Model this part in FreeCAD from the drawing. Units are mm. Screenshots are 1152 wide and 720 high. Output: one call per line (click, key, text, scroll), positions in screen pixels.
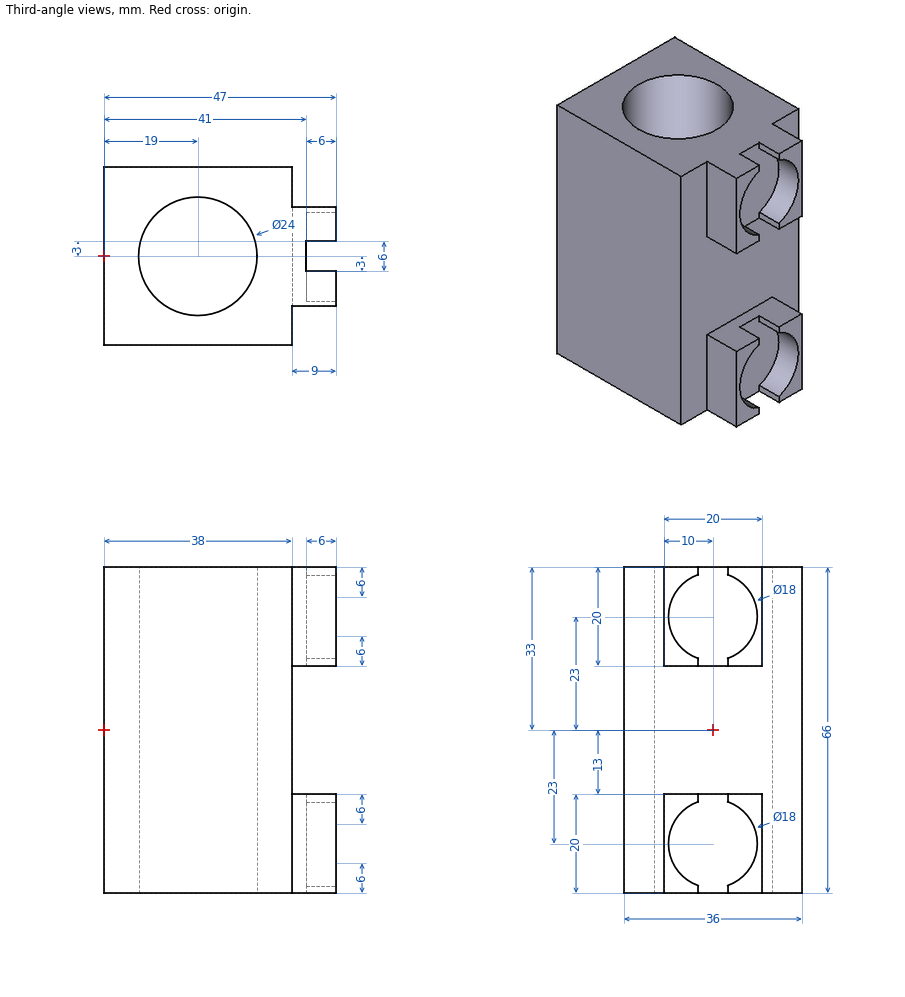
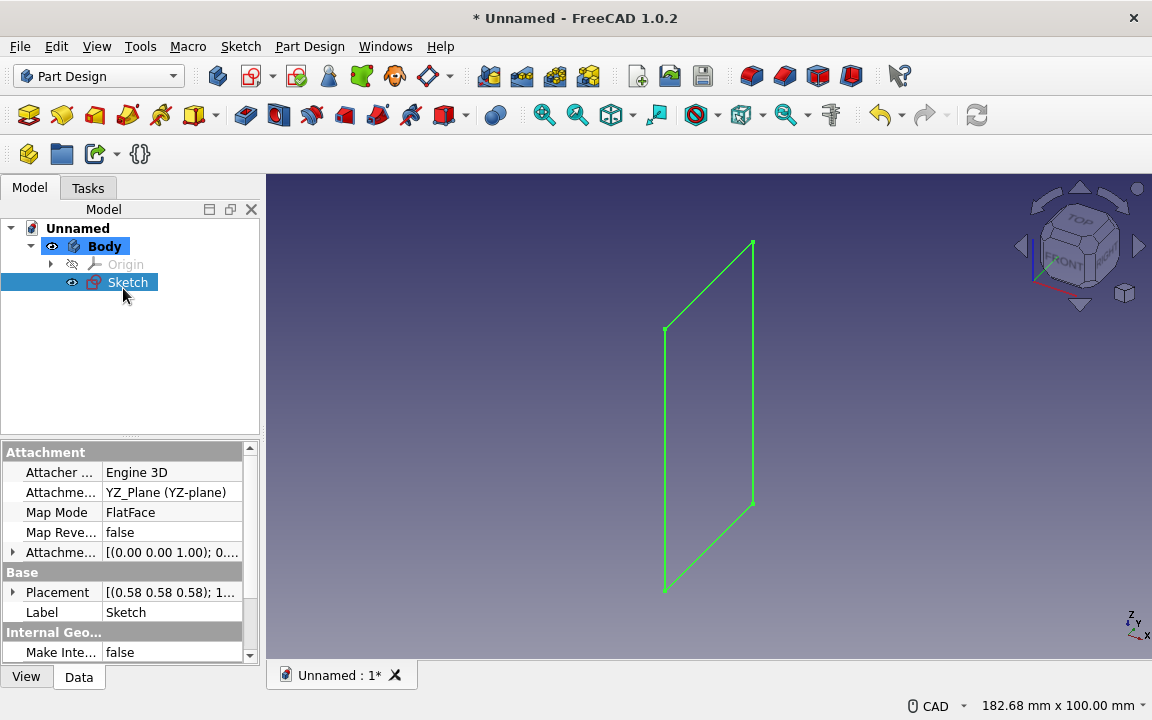
click(29, 116)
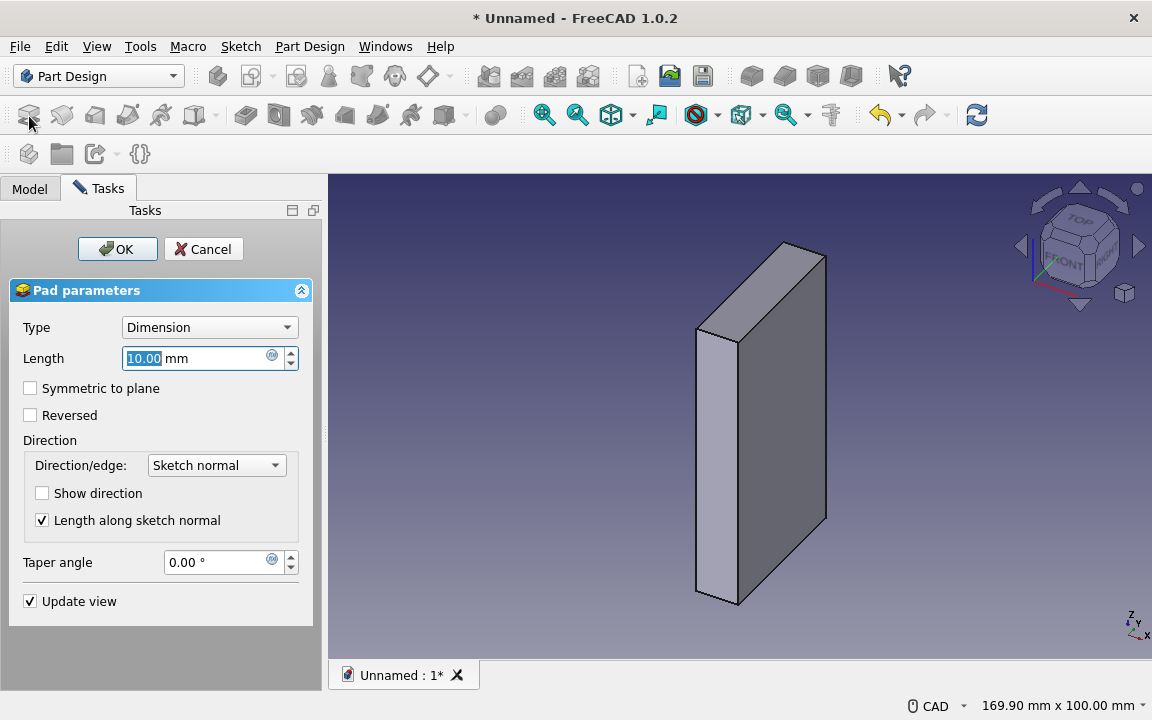
text(38)
key(Tab)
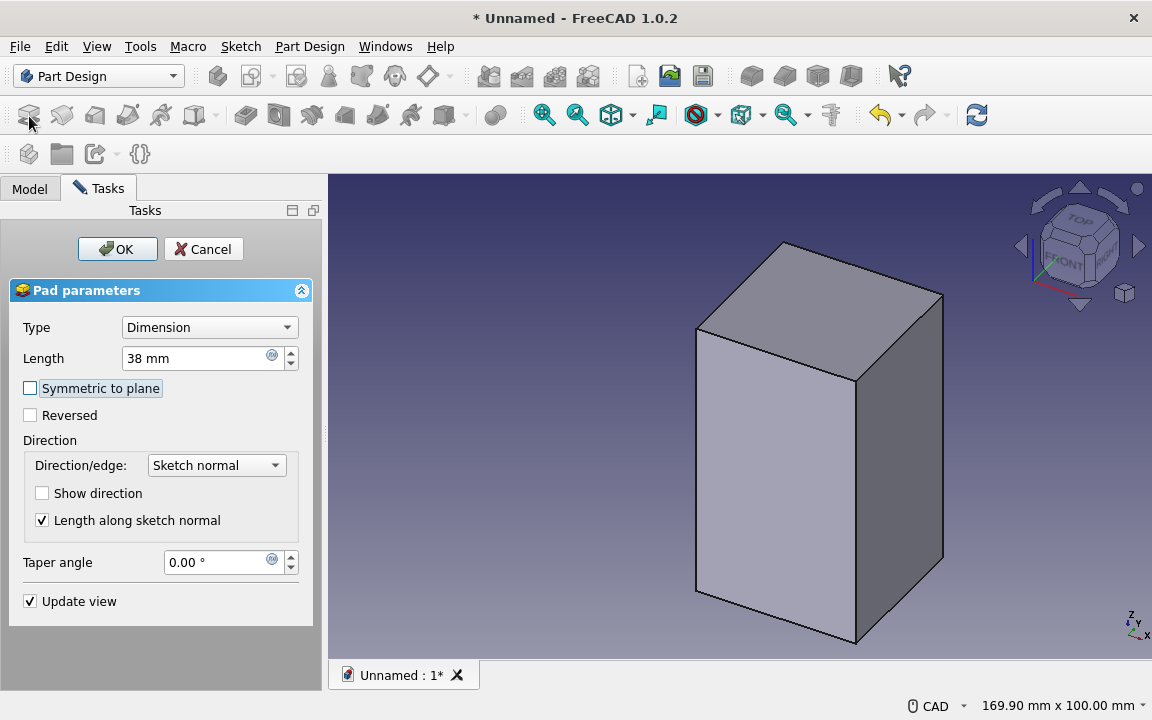
click(118, 249)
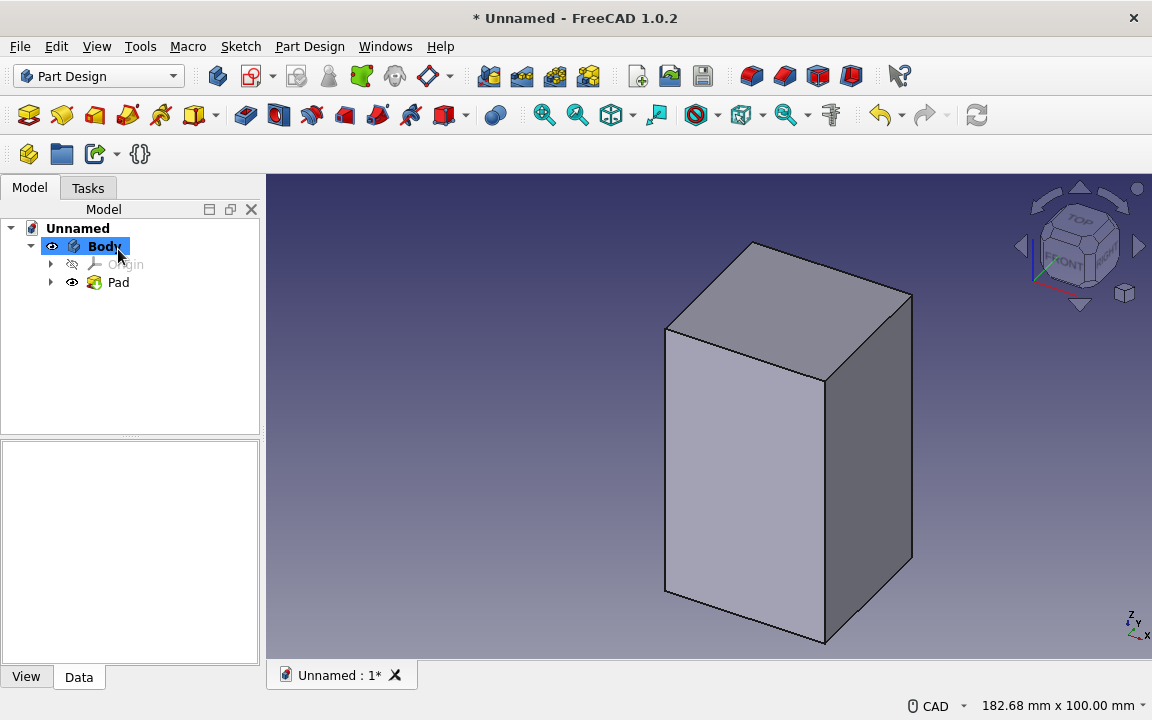
click(869, 431)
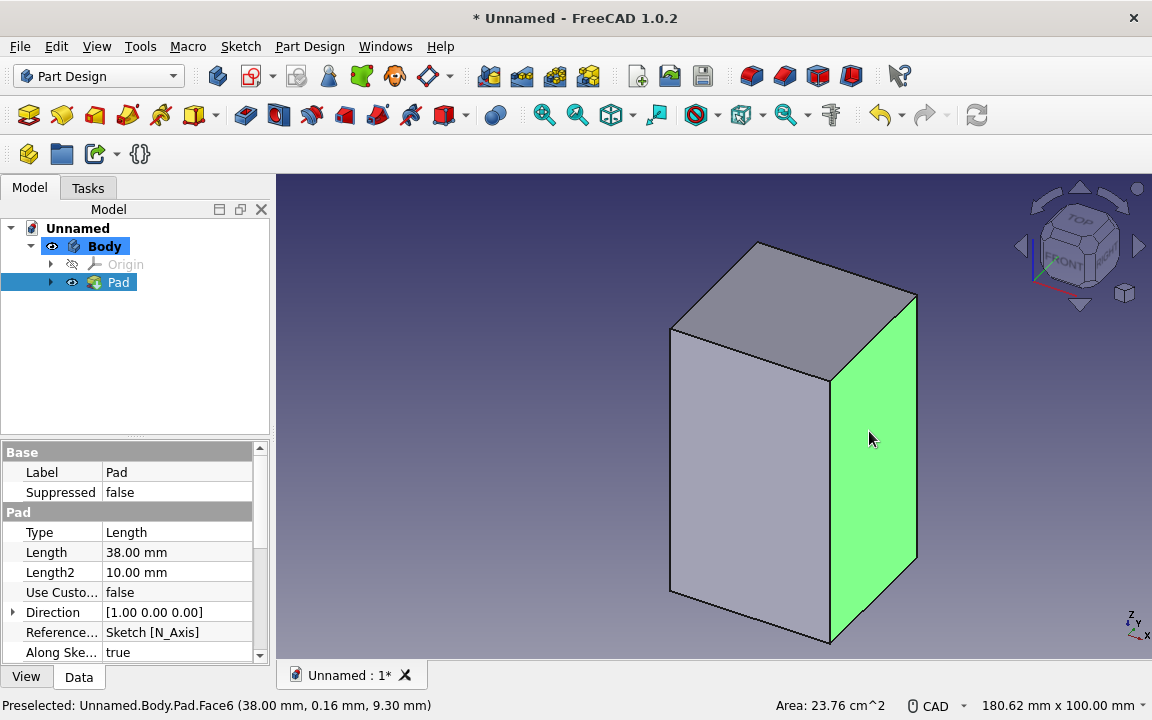
click(250, 76)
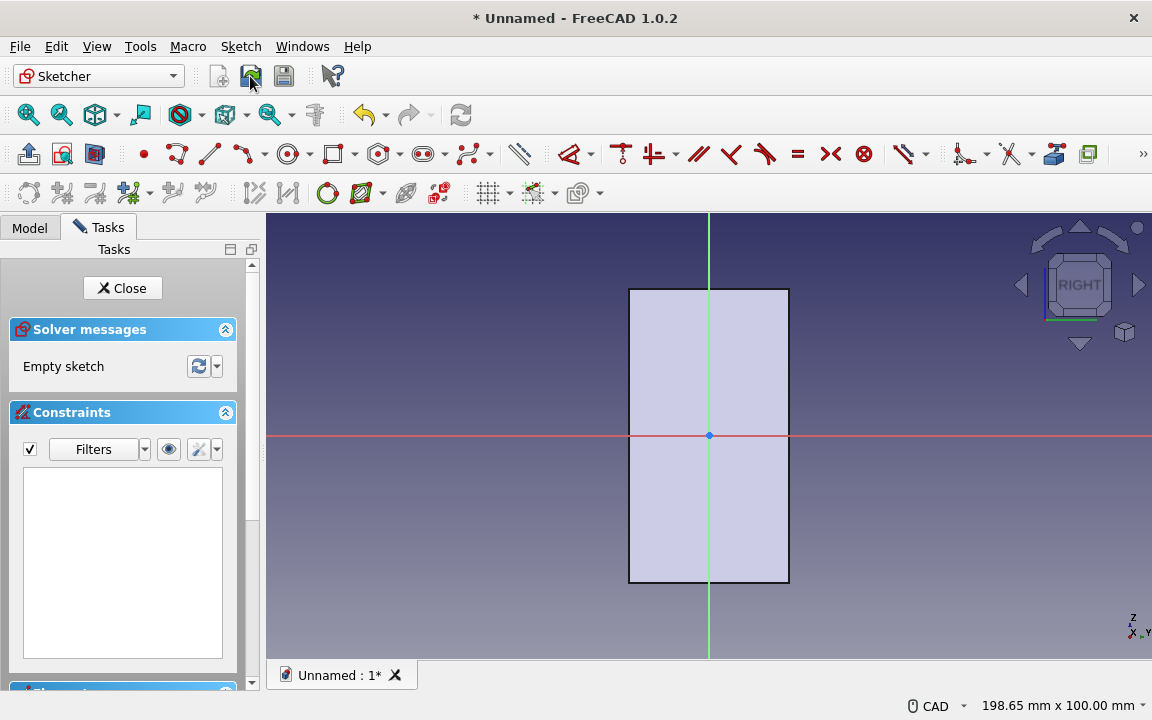
click(332, 154)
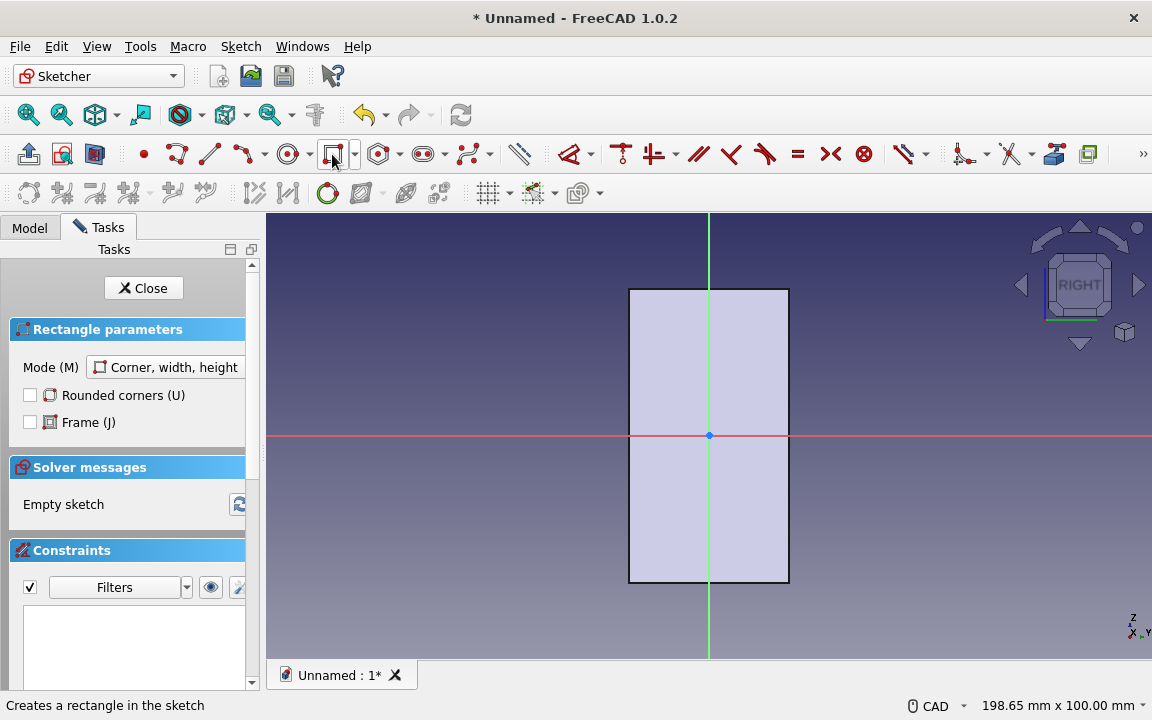
click(664, 289)
click(754, 378)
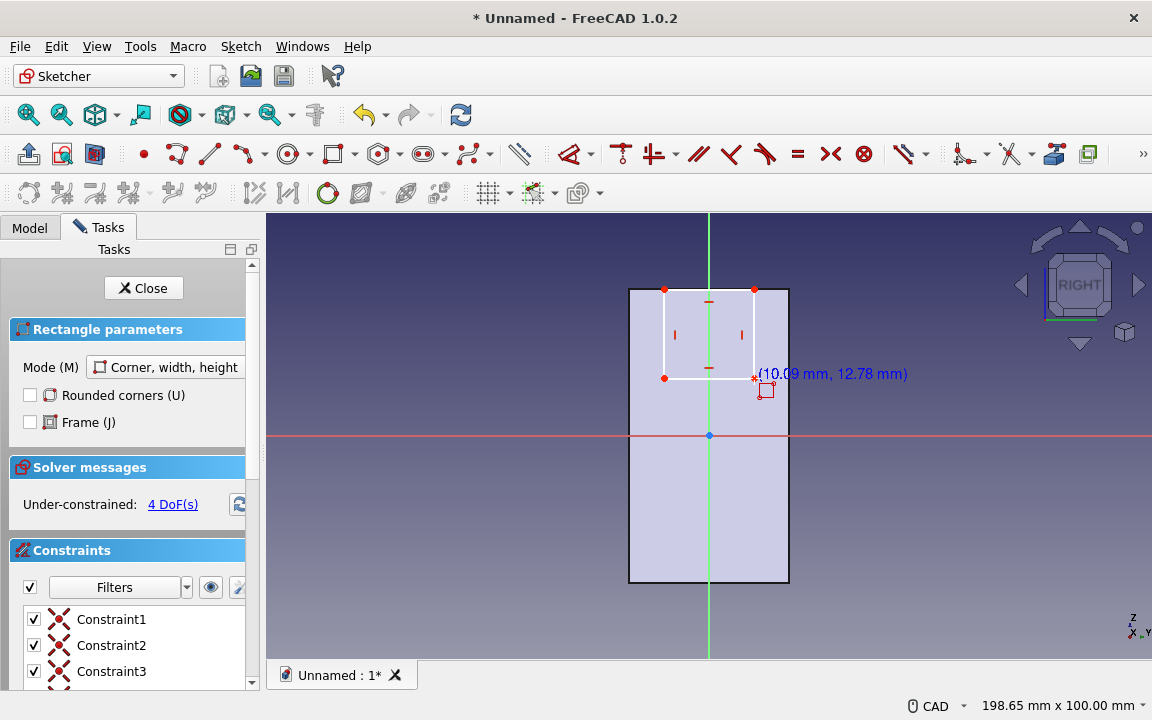
click(664, 494)
click(754, 583)
key(Escape)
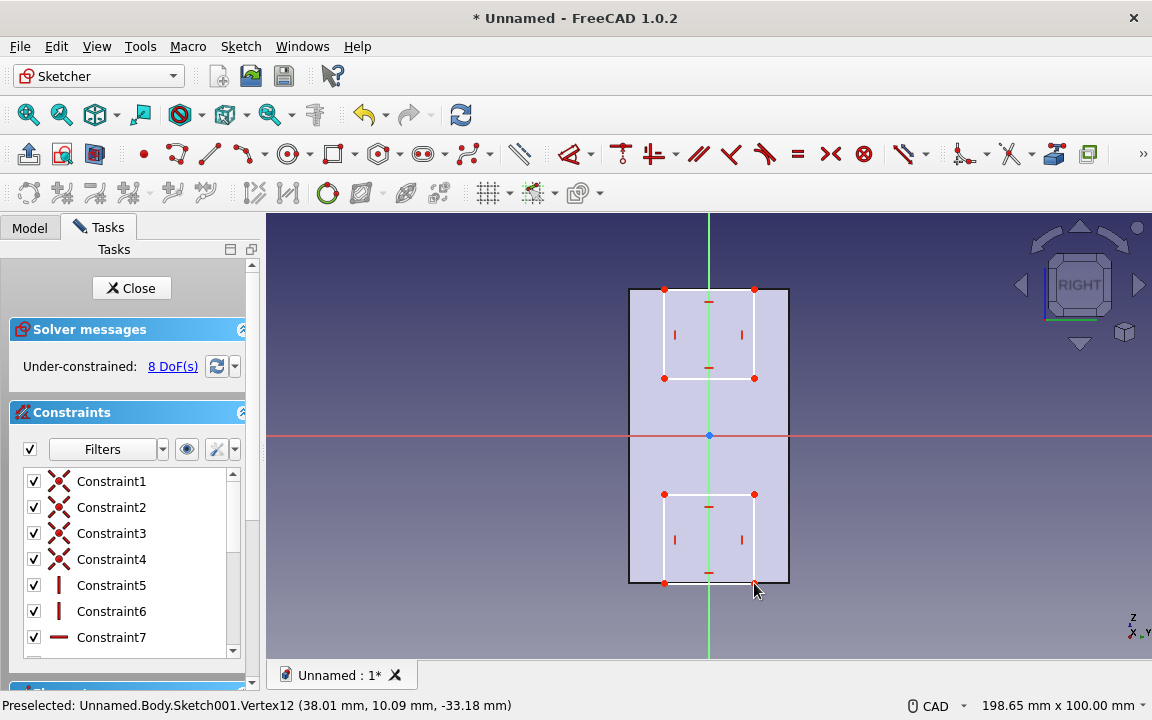
click(568, 154)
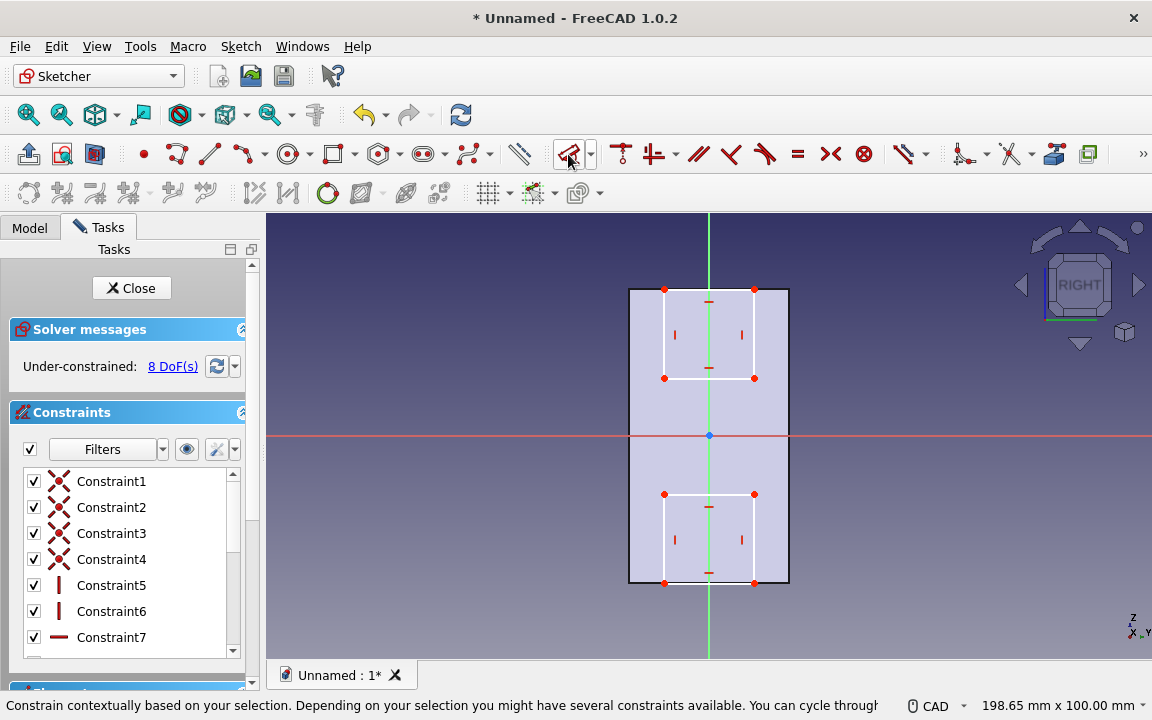
click(664, 317)
click(630, 335)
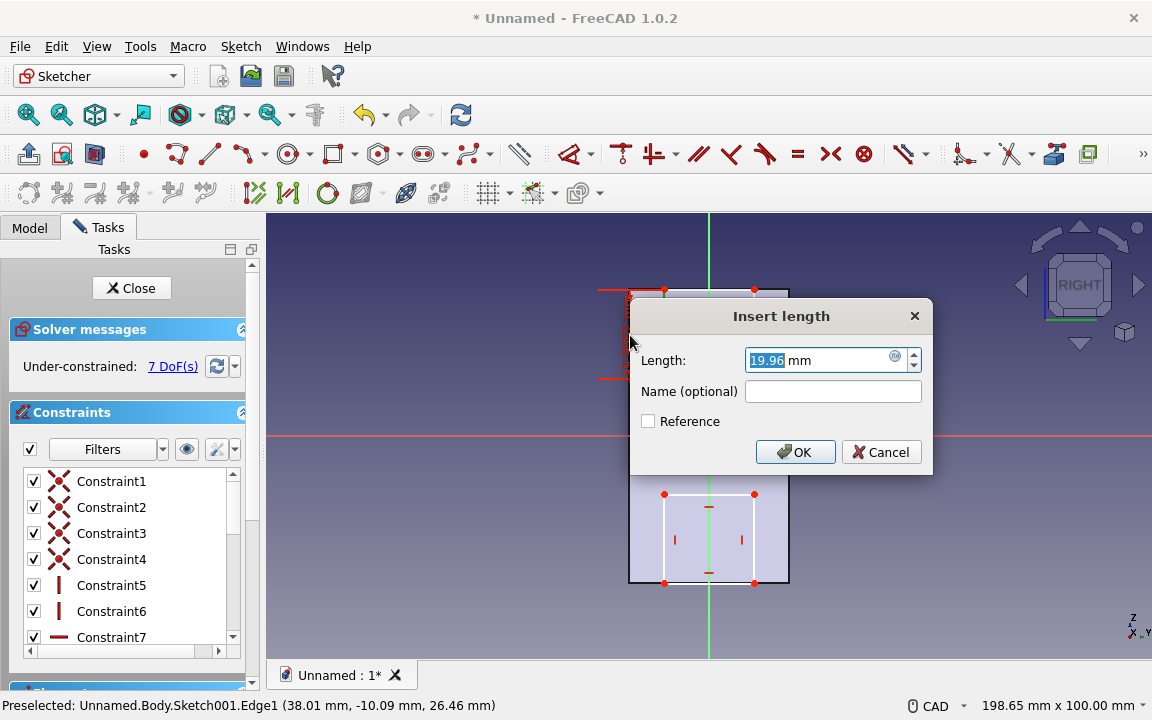
text(20)
key(Return)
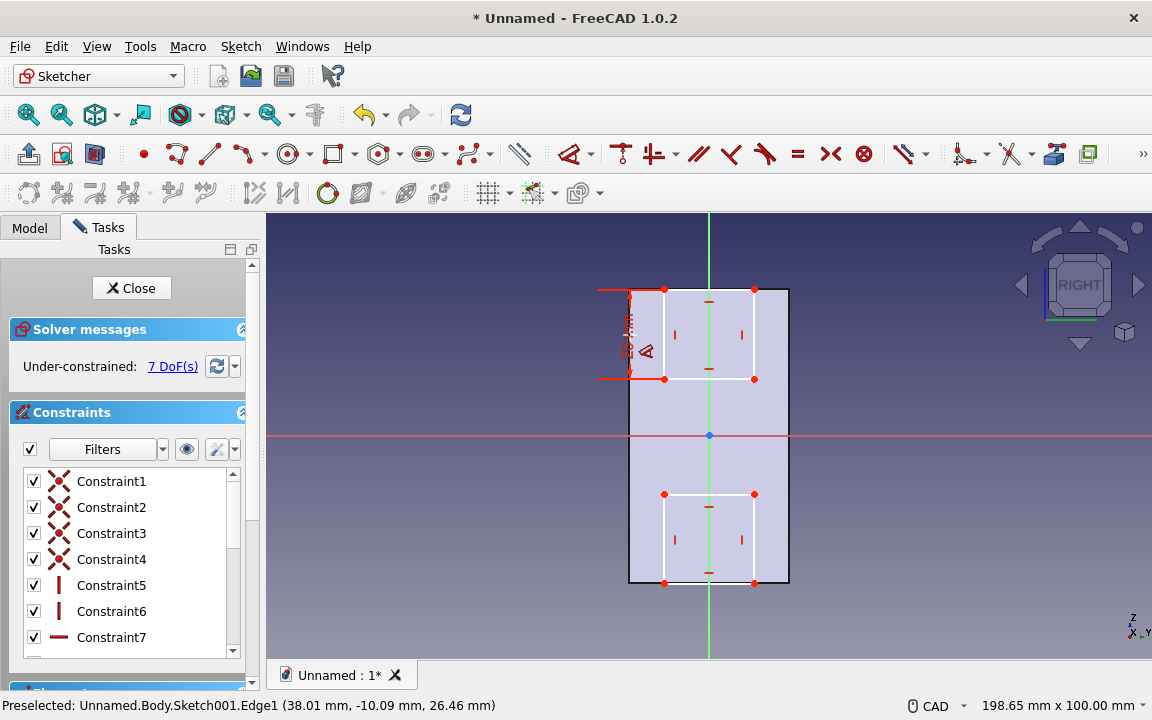
click(691, 379)
click(730, 345)